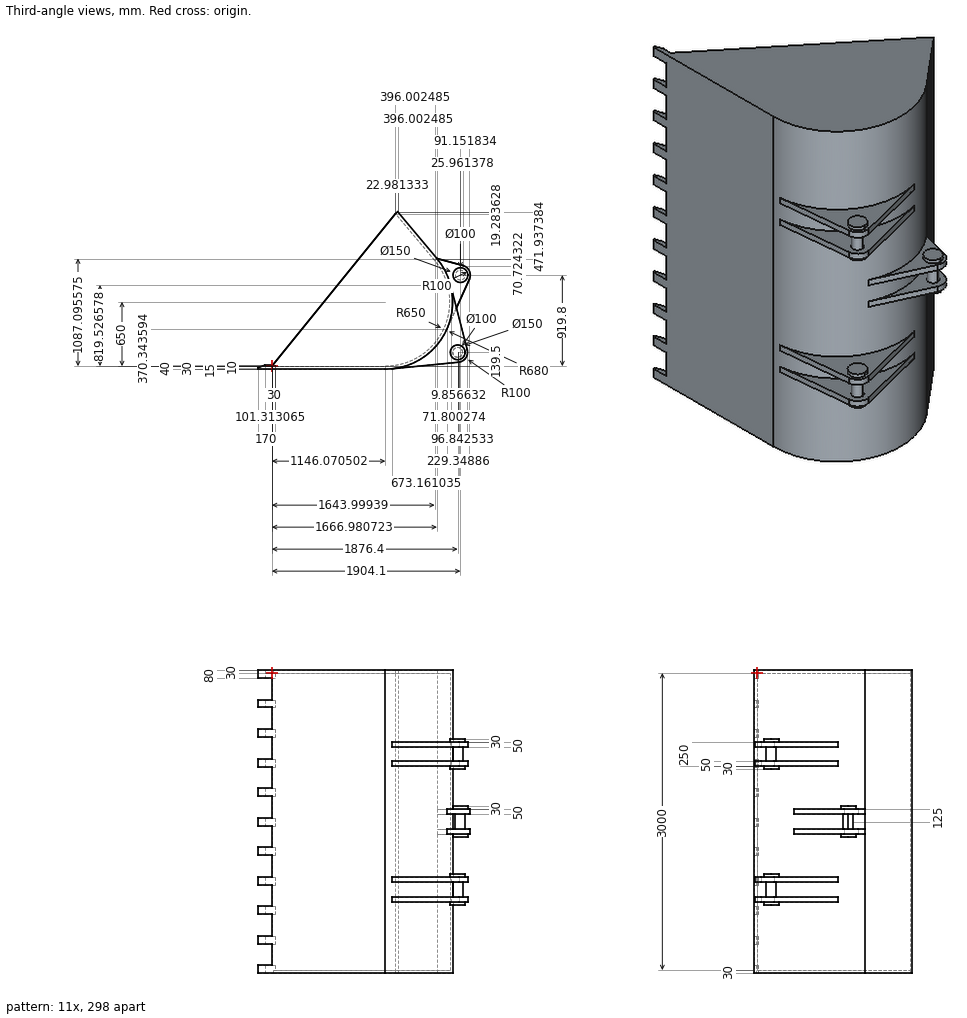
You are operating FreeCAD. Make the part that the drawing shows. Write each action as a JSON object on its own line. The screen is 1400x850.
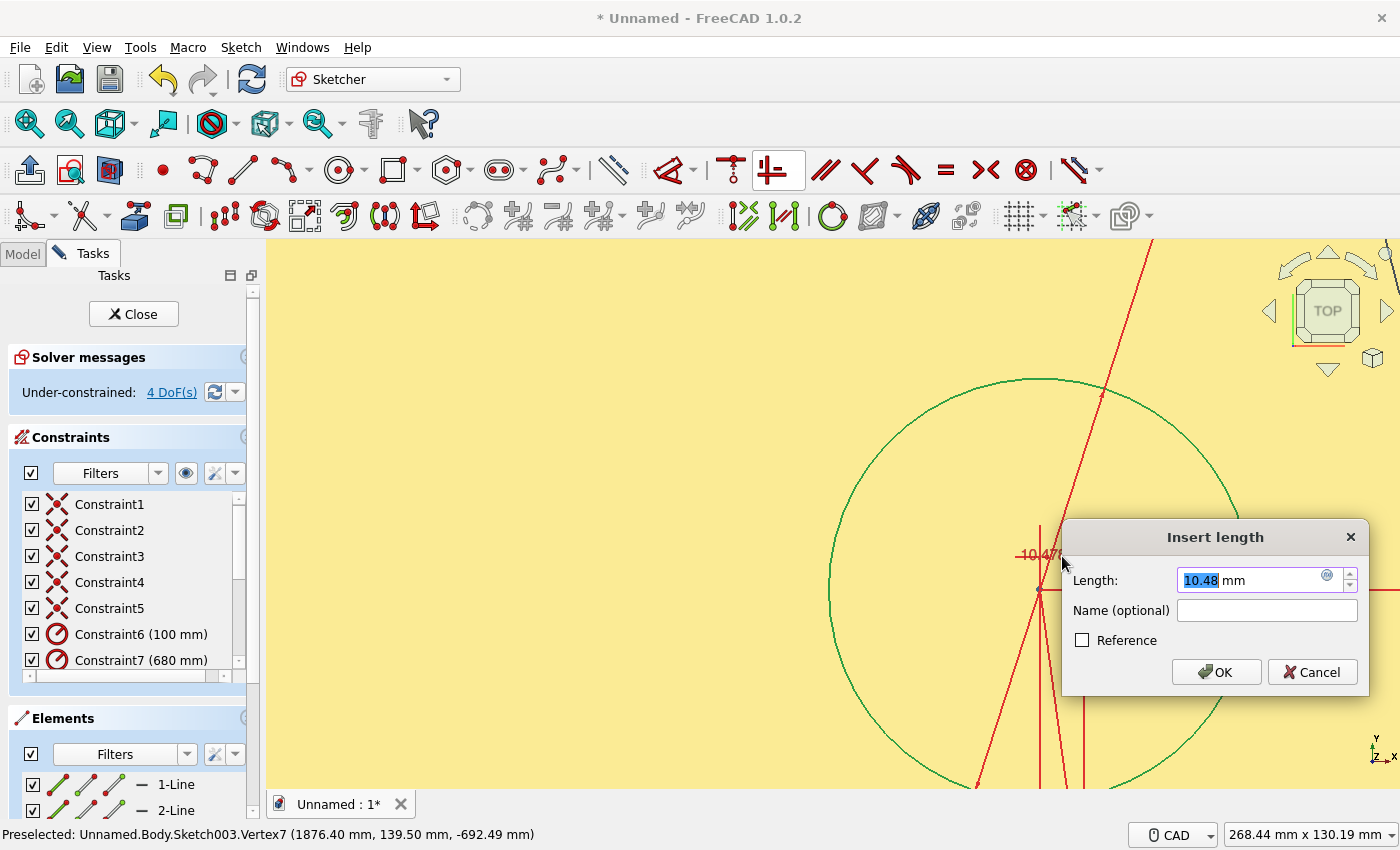
{"action": "type", "text": "9.856632"}
{"action": "key", "text": "Return"}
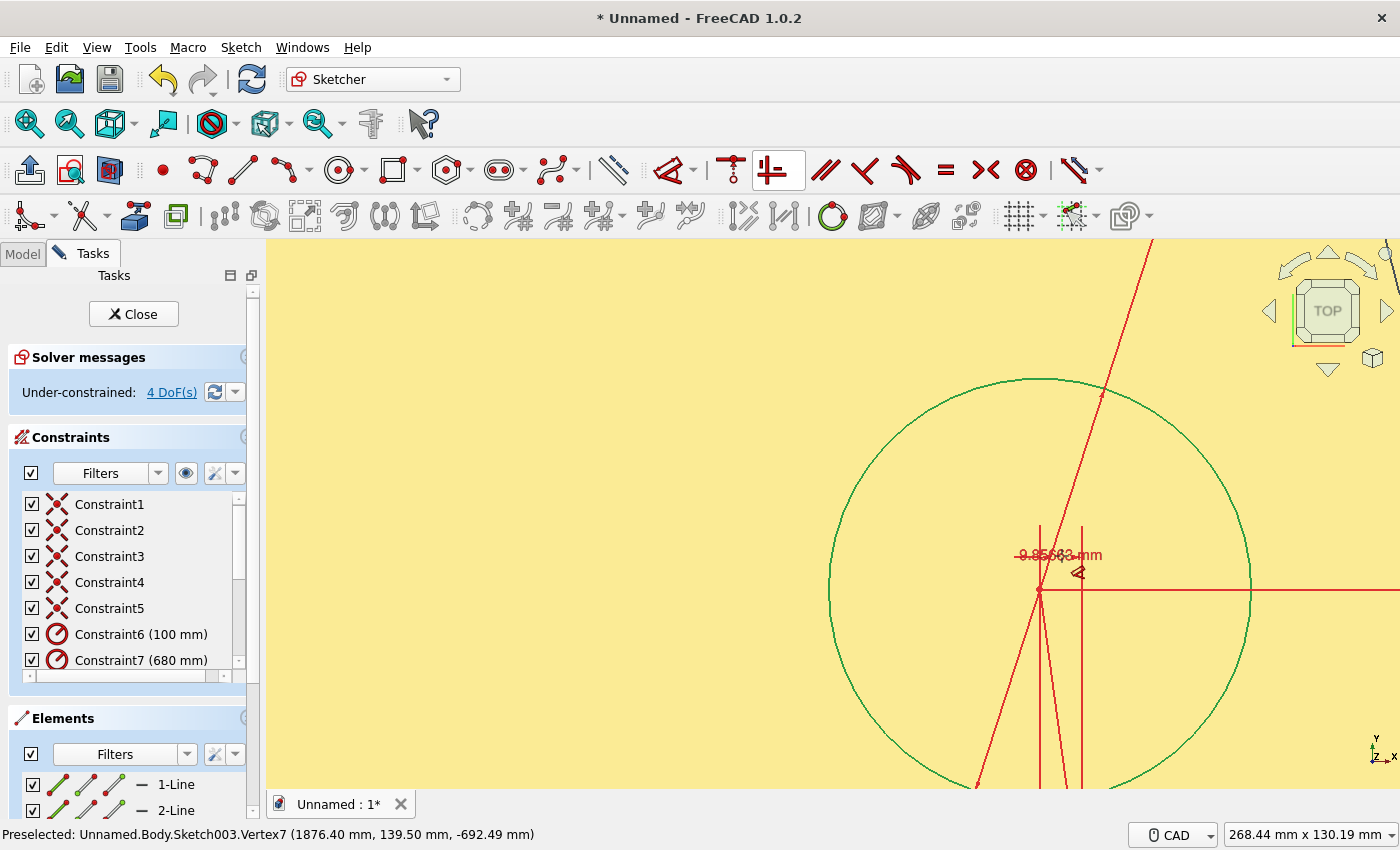
{"action": "scroll", "coordinate": [1044, 595], "scroll_direction": "down", "scroll_amount": 13}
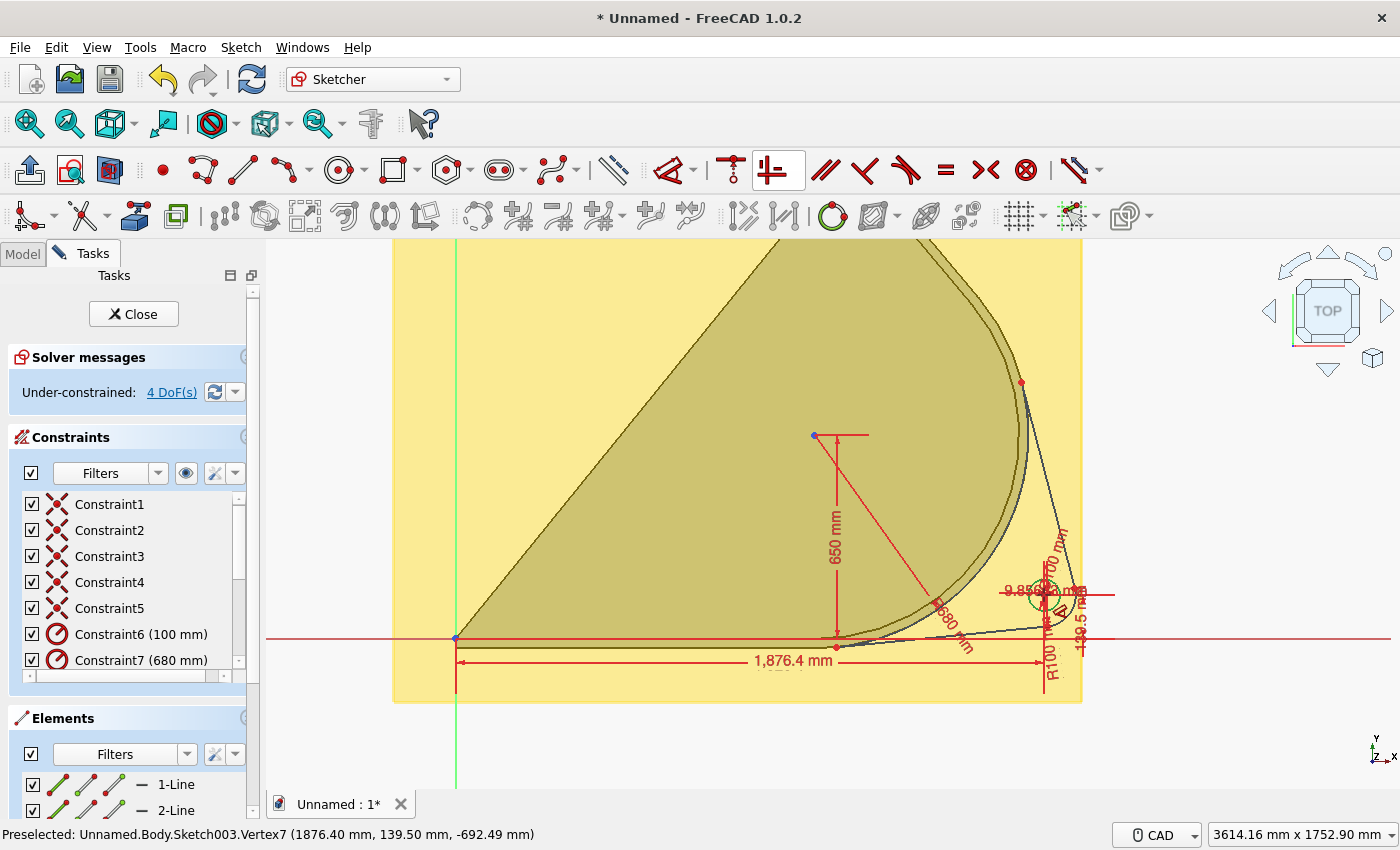
{"action": "scroll", "coordinate": [1075, 588], "scroll_direction": "up", "scroll_amount": 2}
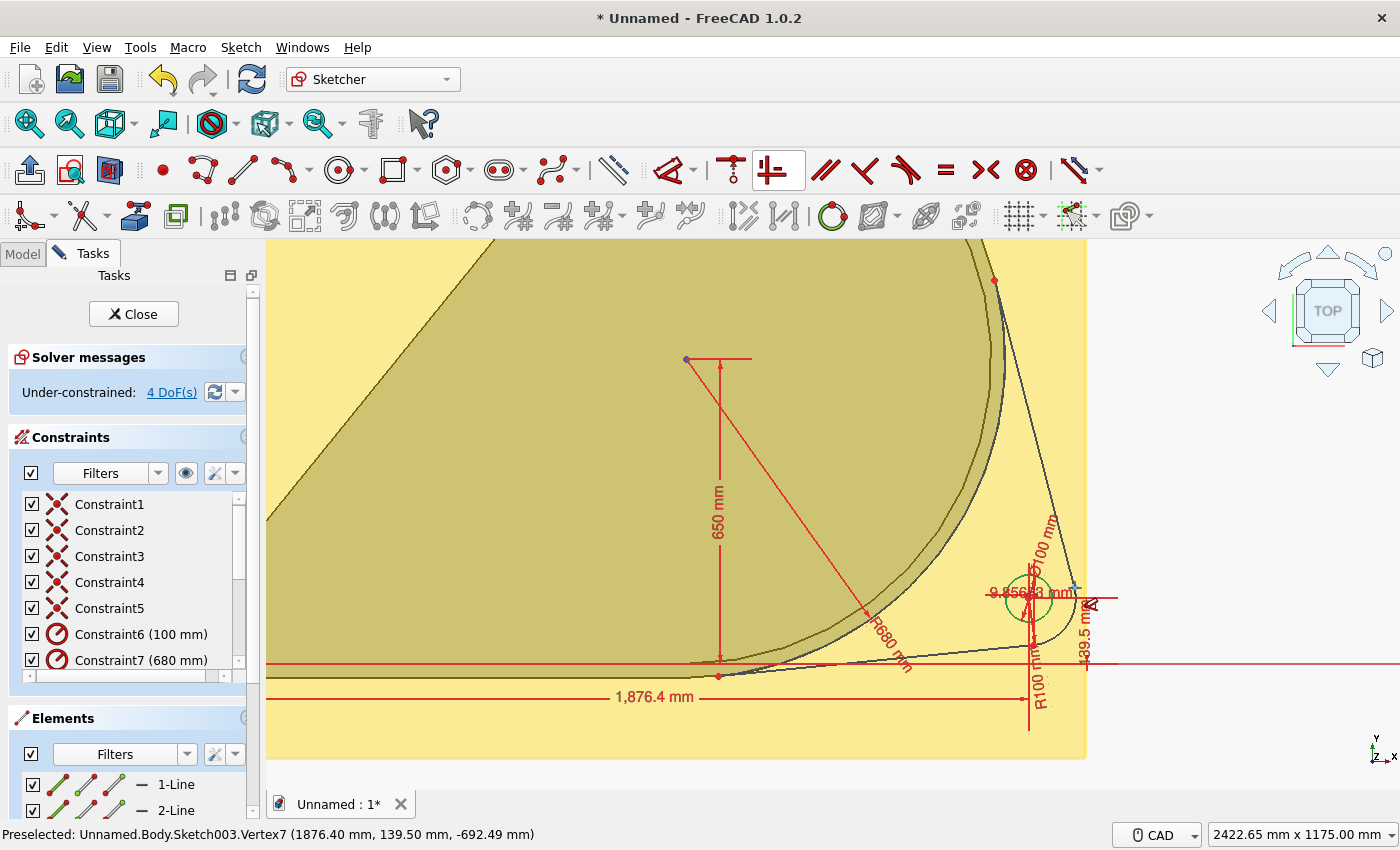
{"action": "left_click", "coordinate": [1074, 588]}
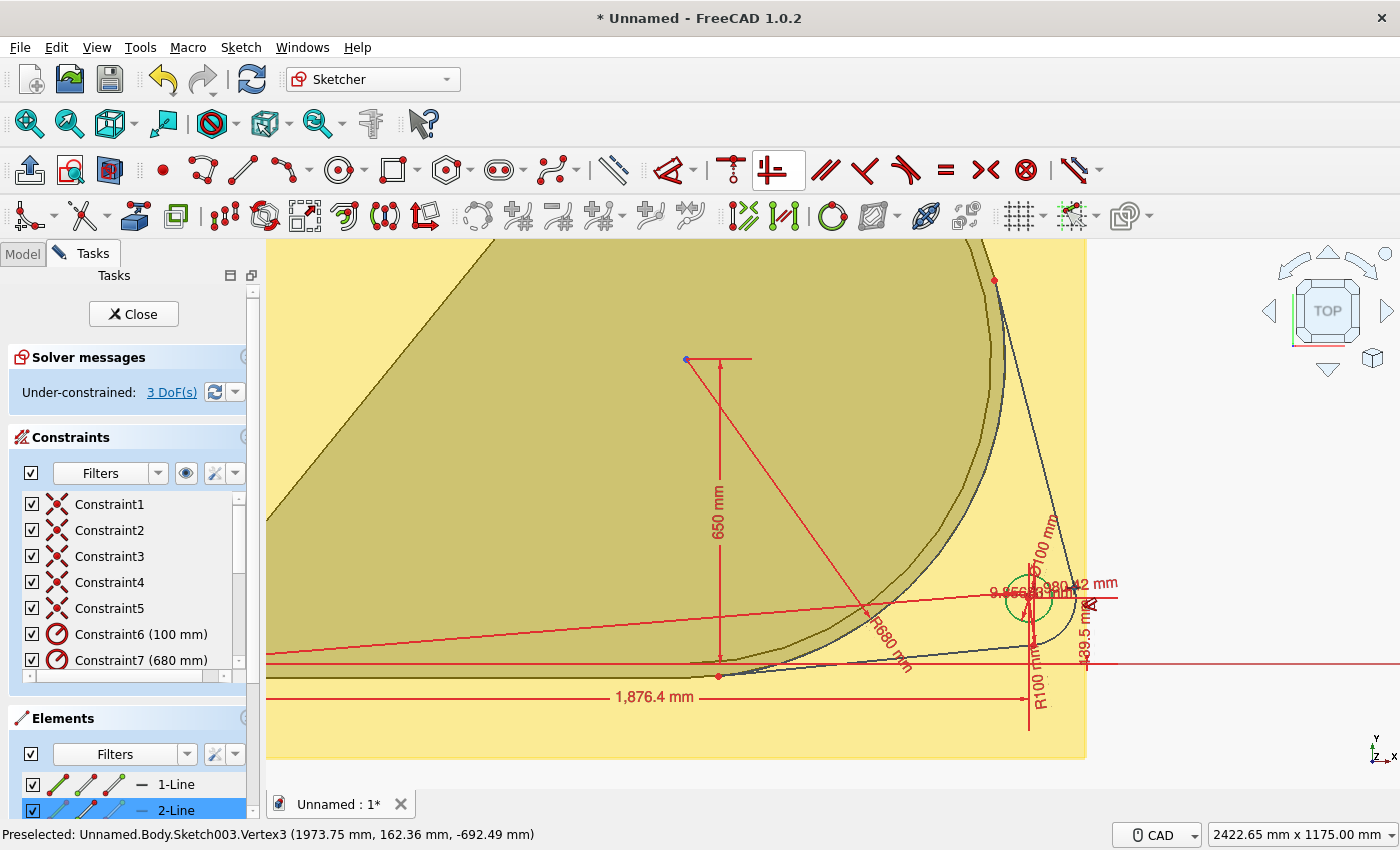
{"action": "left_click", "coordinate": [1029, 598]}
{"action": "left_click", "coordinate": [1036, 506]}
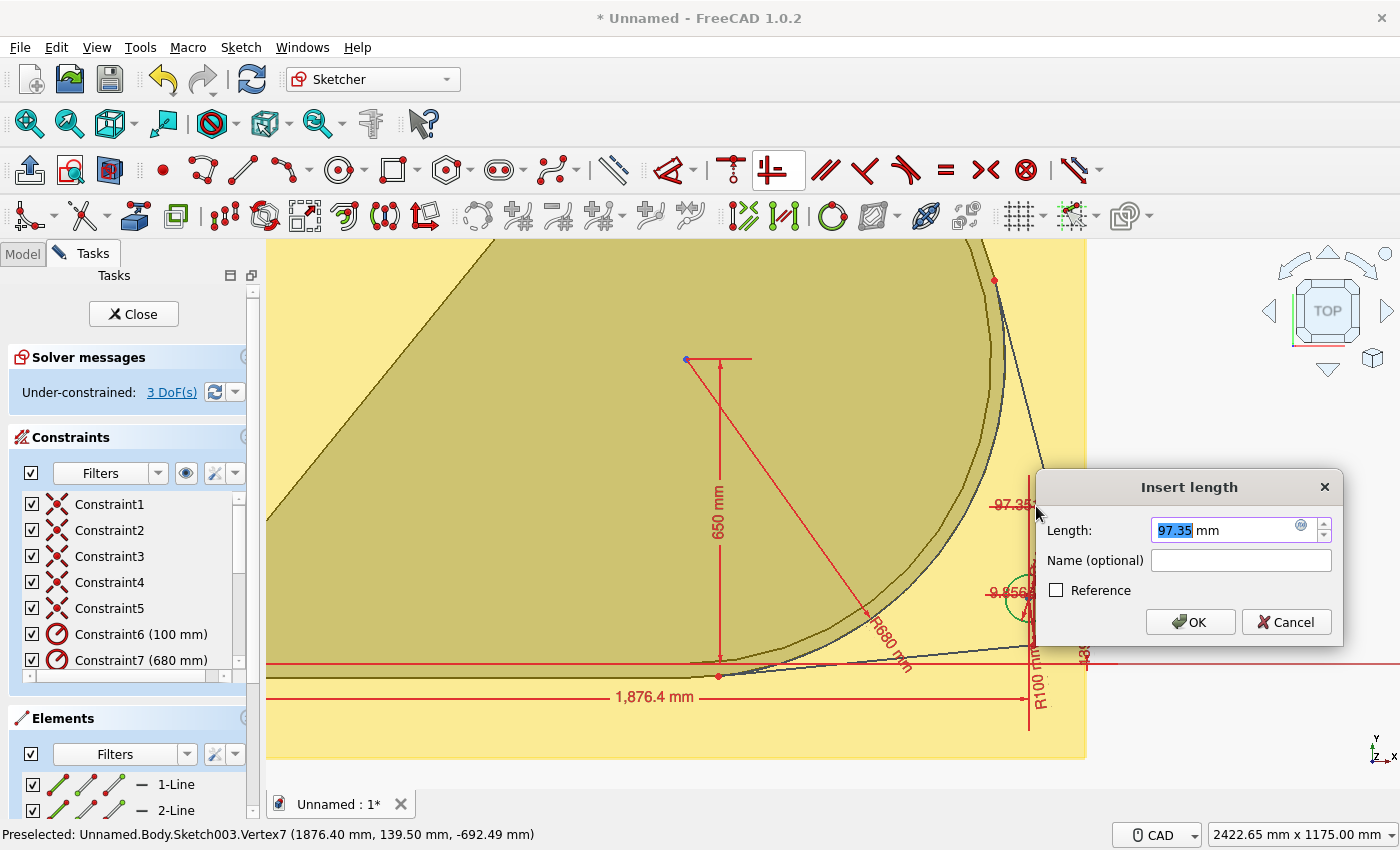
{"action": "type", "text": "96.842533"}
{"action": "key", "text": "Return"}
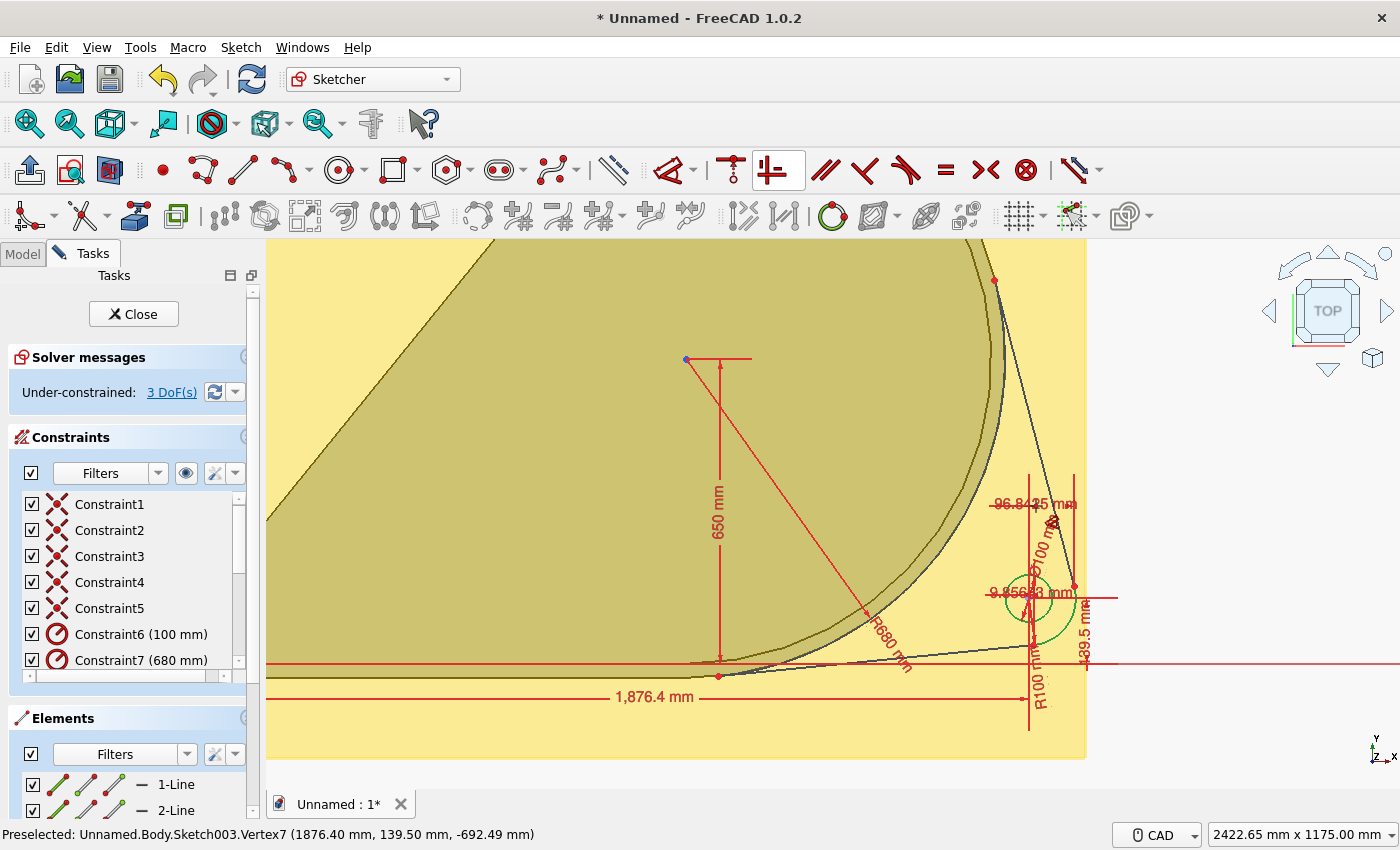
{"action": "left_click", "coordinate": [995, 281]}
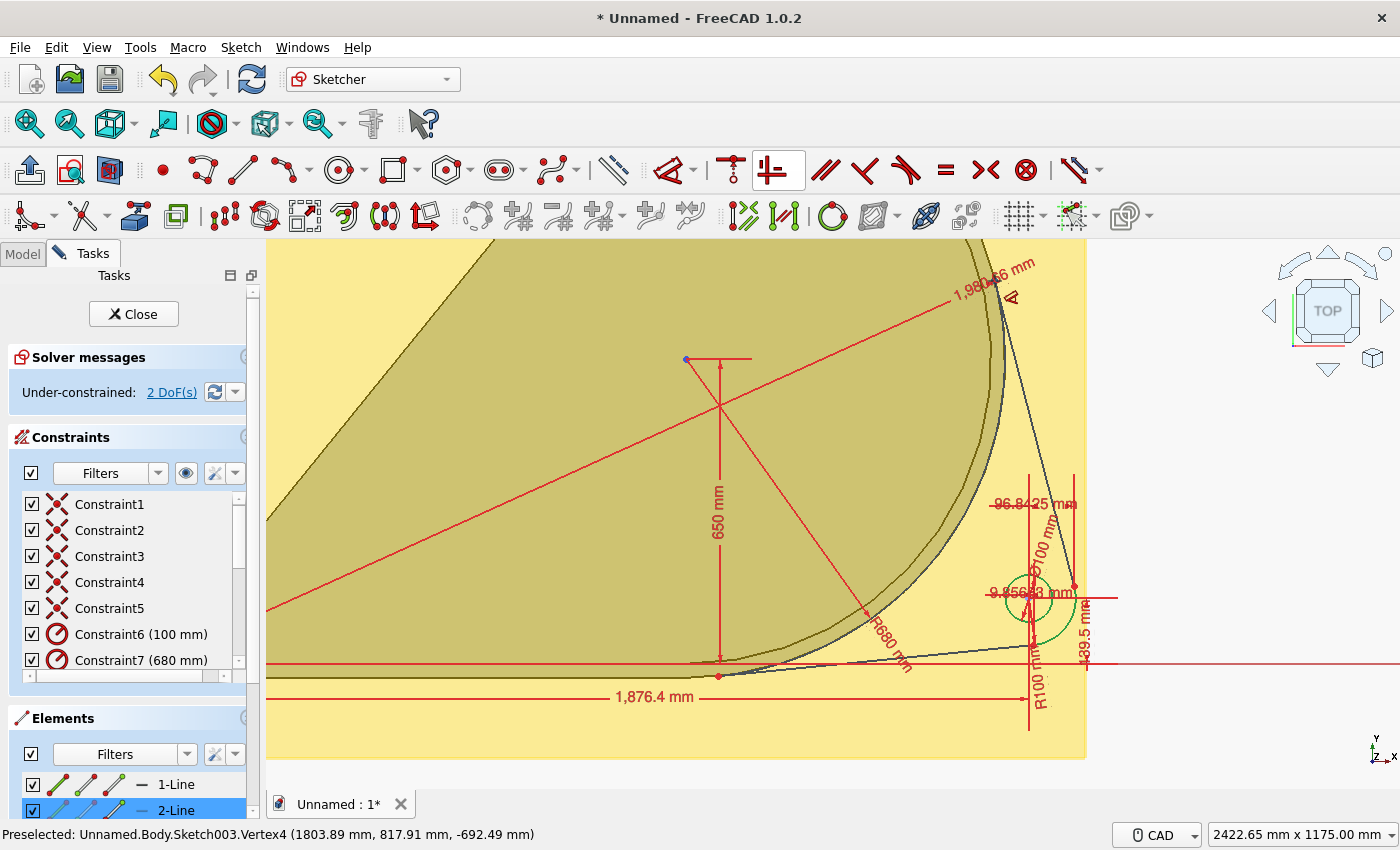
{"action": "left_click", "coordinate": [1029, 598]}
{"action": "left_click", "coordinate": [1012, 632]}